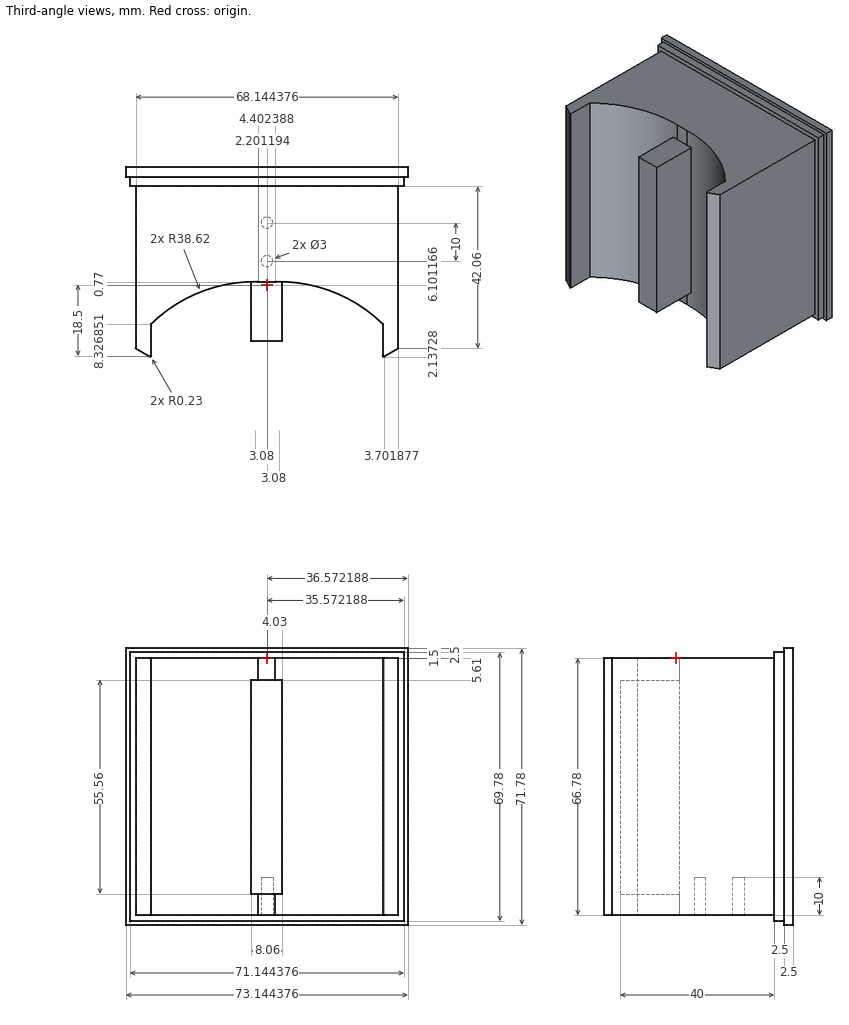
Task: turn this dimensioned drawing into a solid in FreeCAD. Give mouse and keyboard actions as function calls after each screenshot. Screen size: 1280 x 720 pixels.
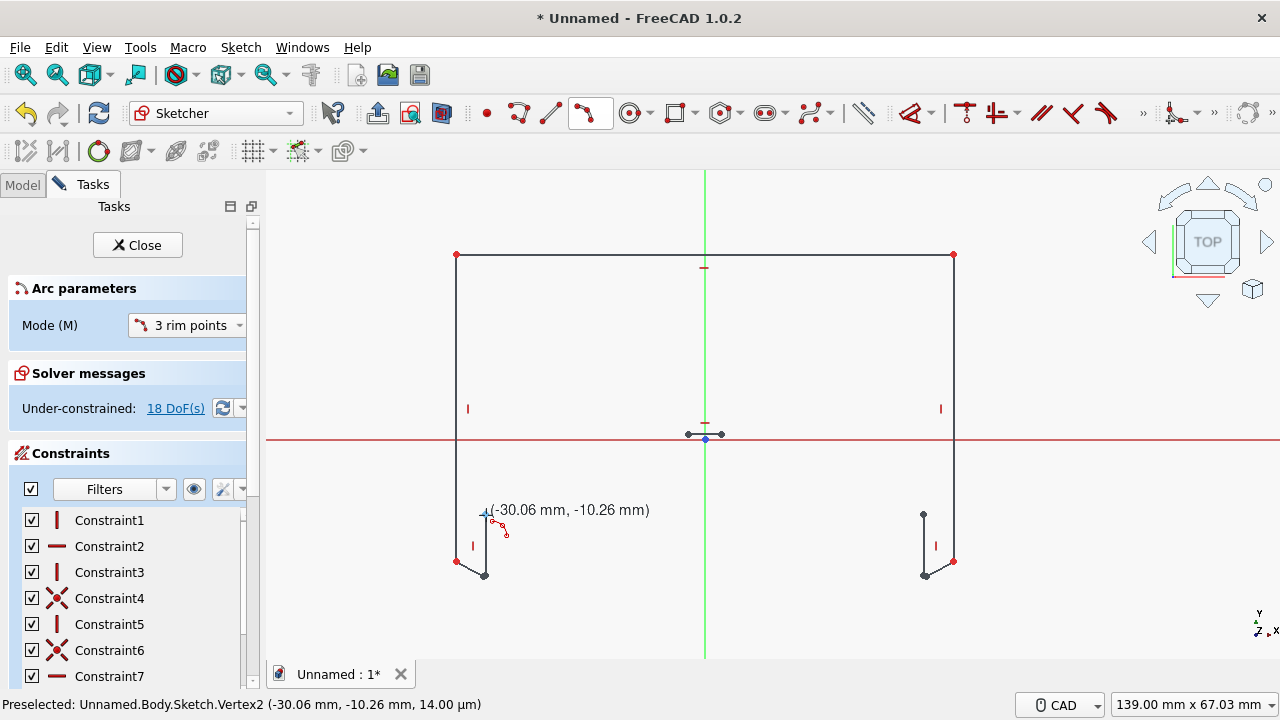
scroll(689, 434, up, 6)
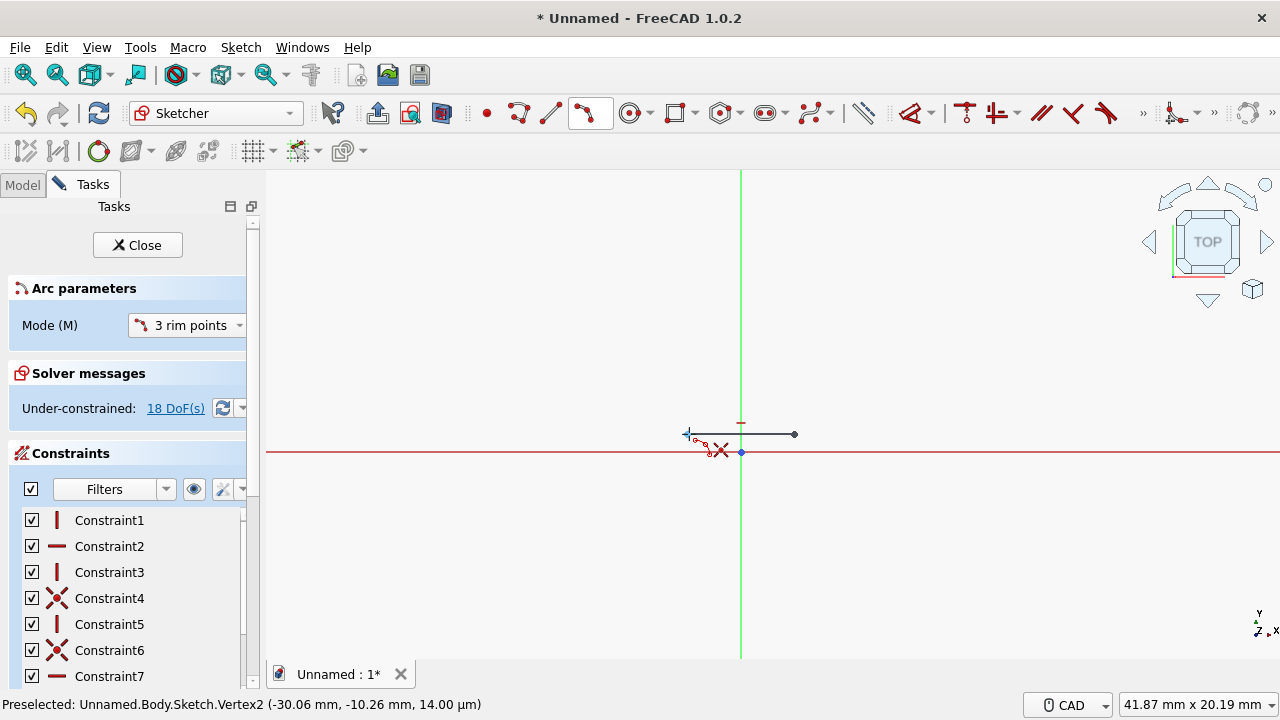
click(688, 434)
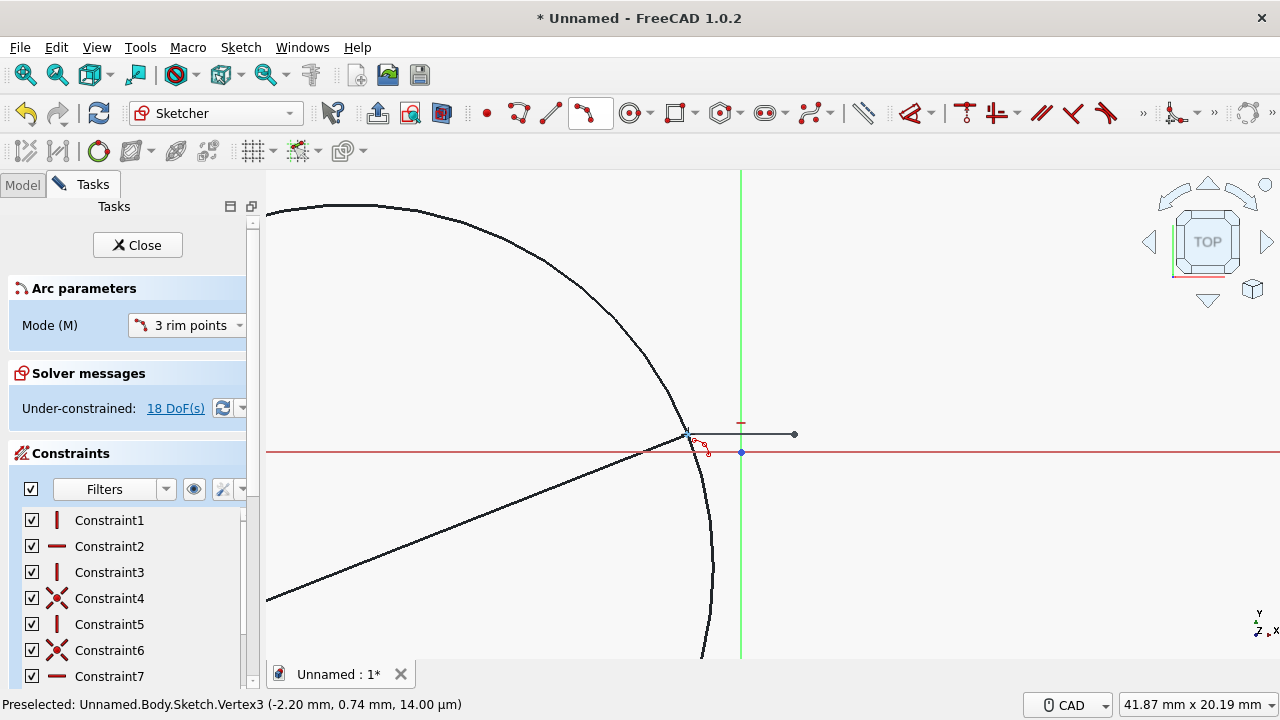
scroll(689, 434, down, 6)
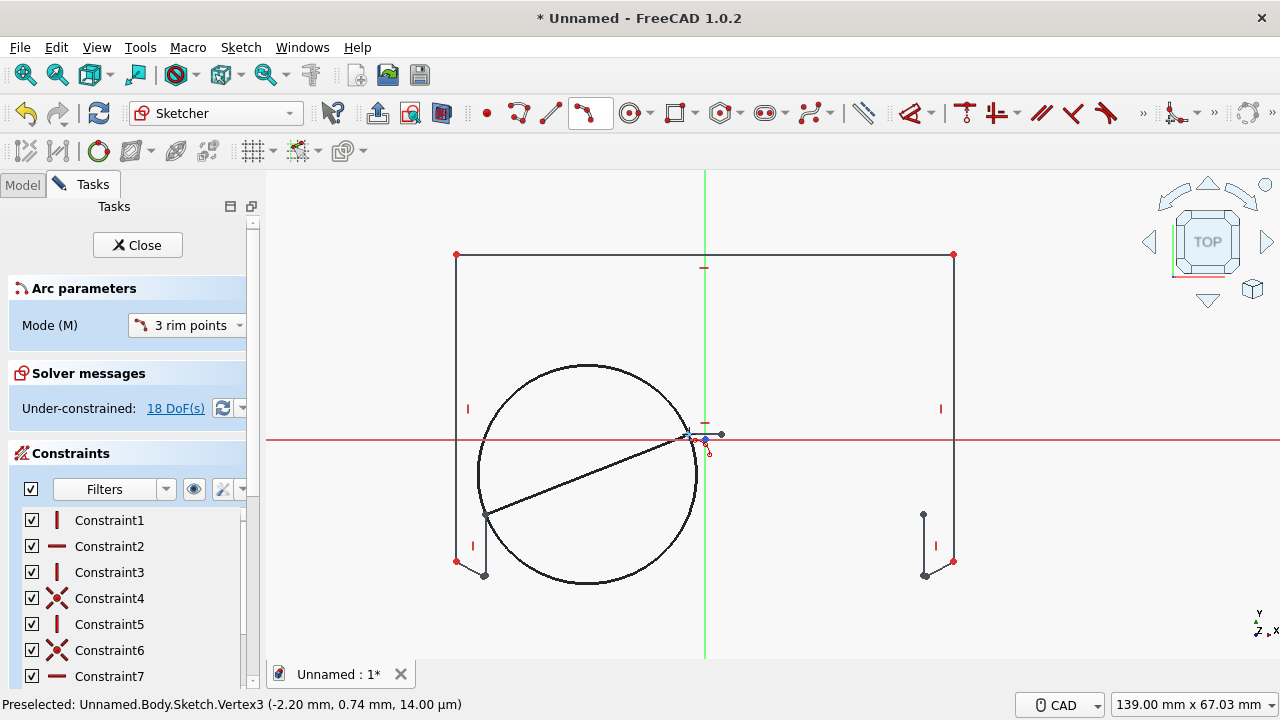
click(559, 463)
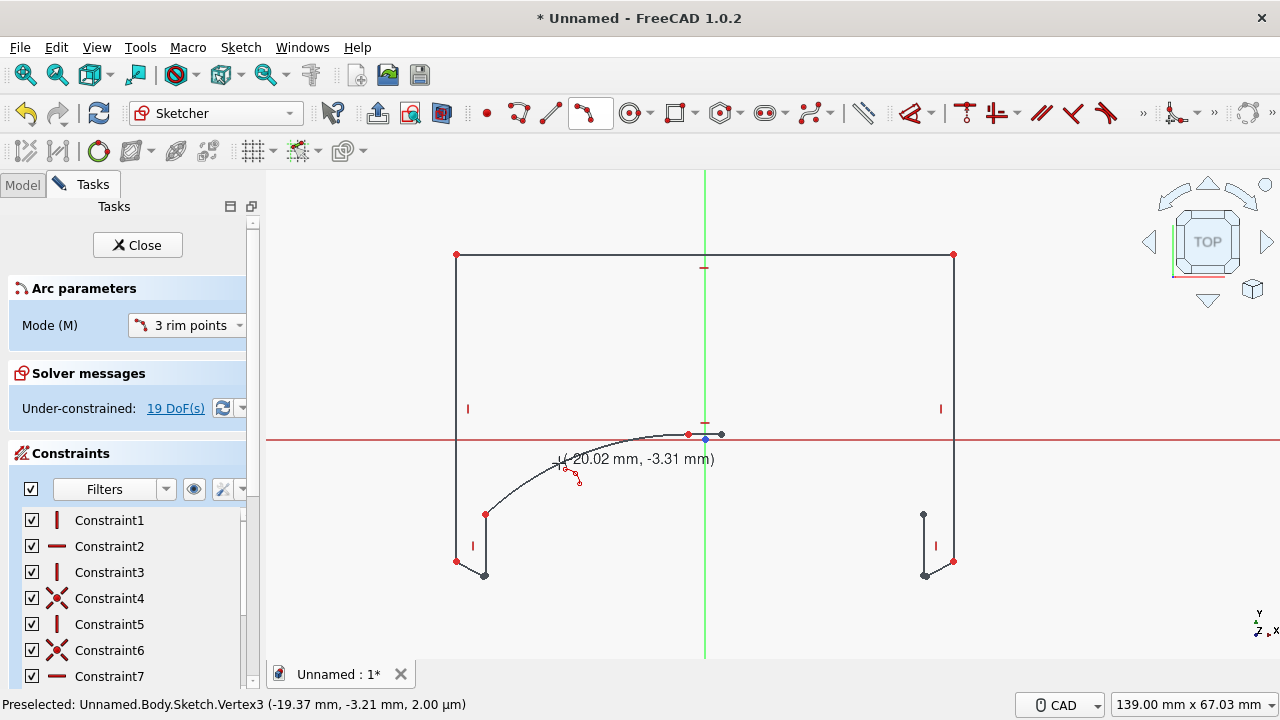
scroll(721, 434, up, 6)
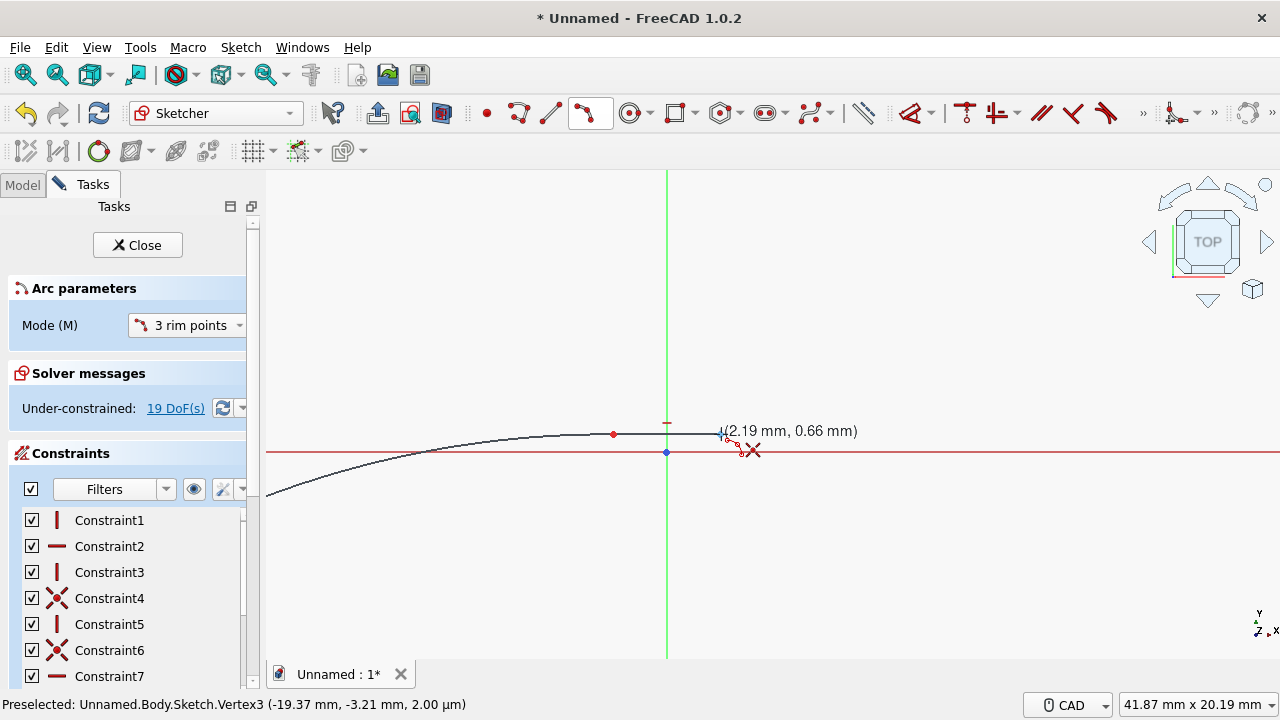
click(721, 434)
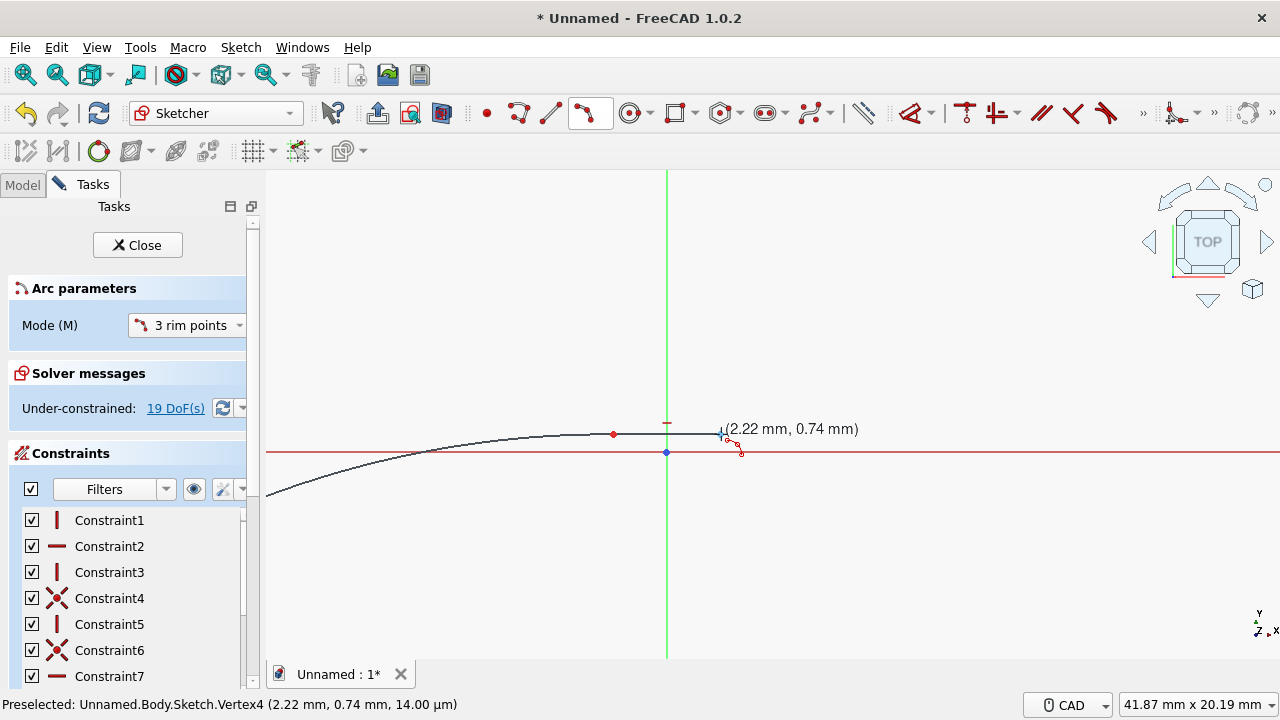
scroll(721, 434, down, 6)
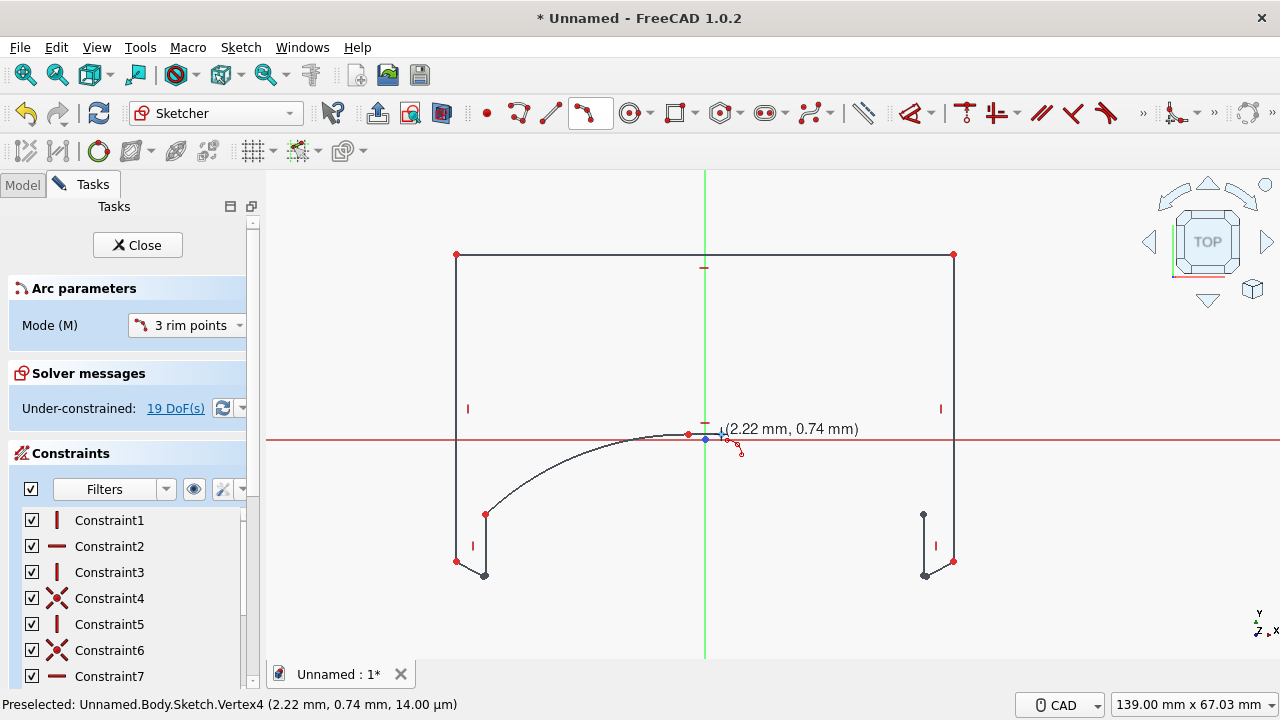
click(924, 515)
click(851, 463)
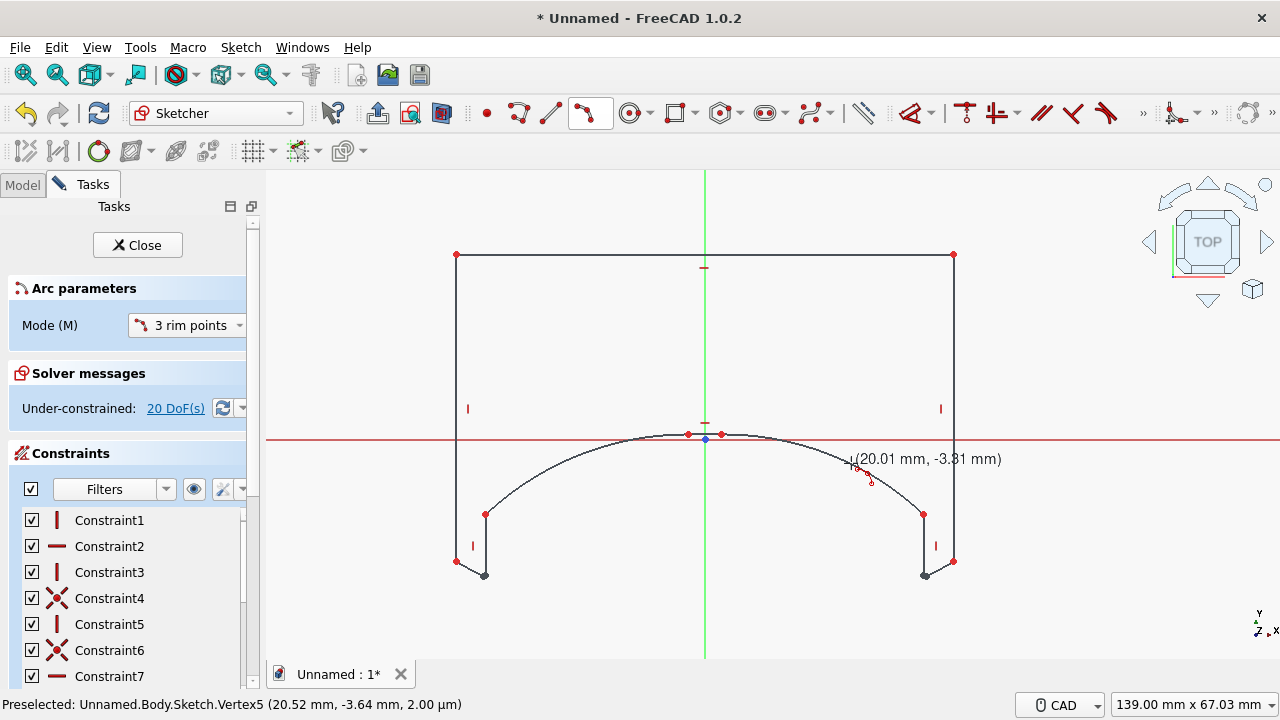
scroll(924, 575, up, 9)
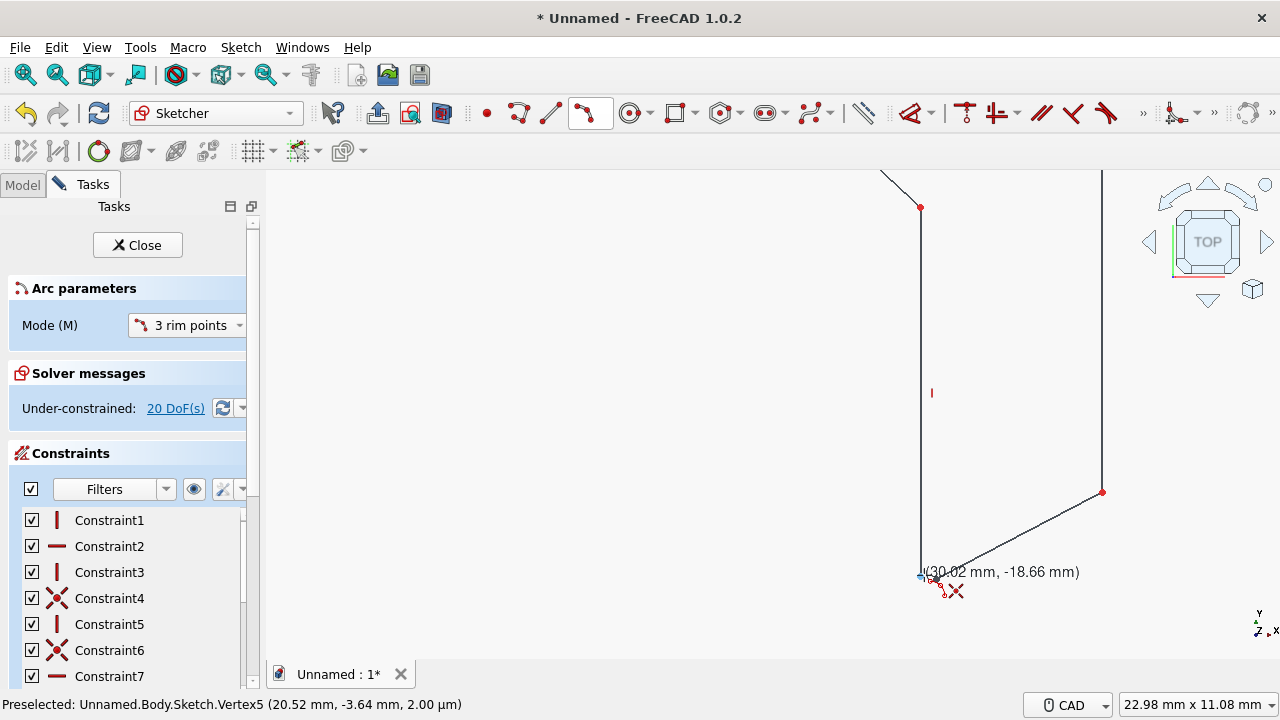
click(921, 577)
click(936, 579)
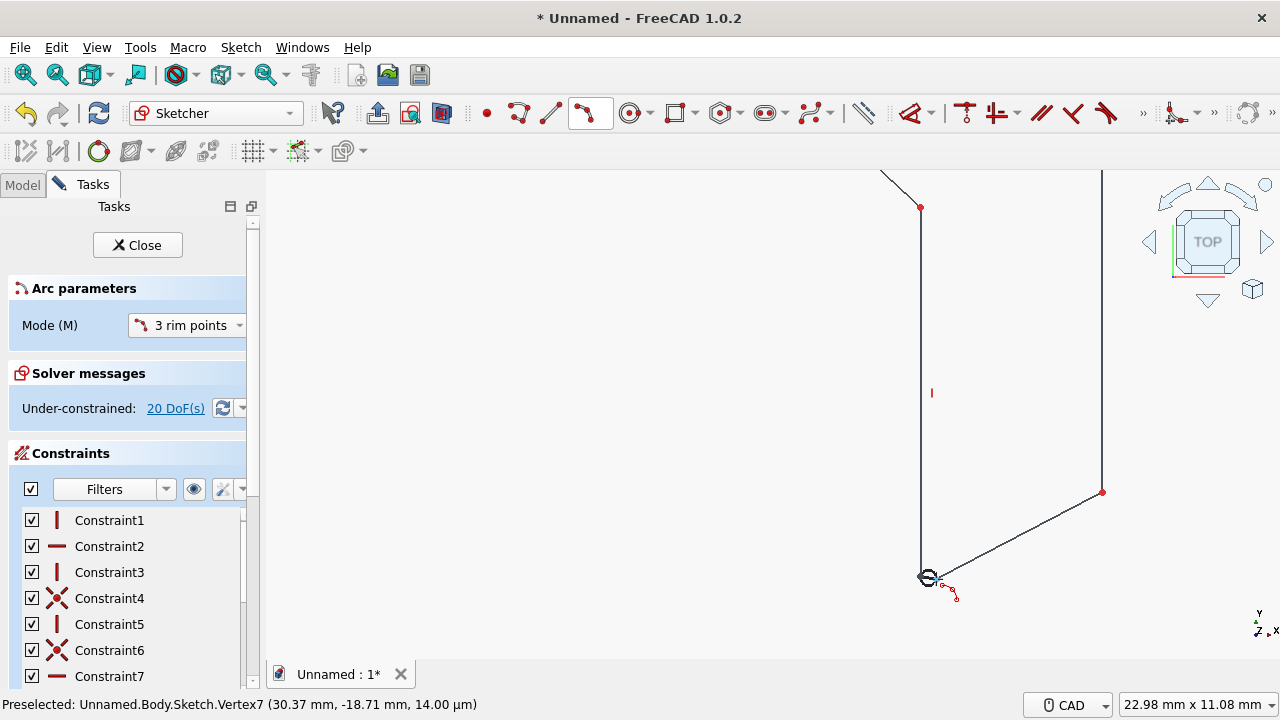
scroll(926, 578, up, 6)